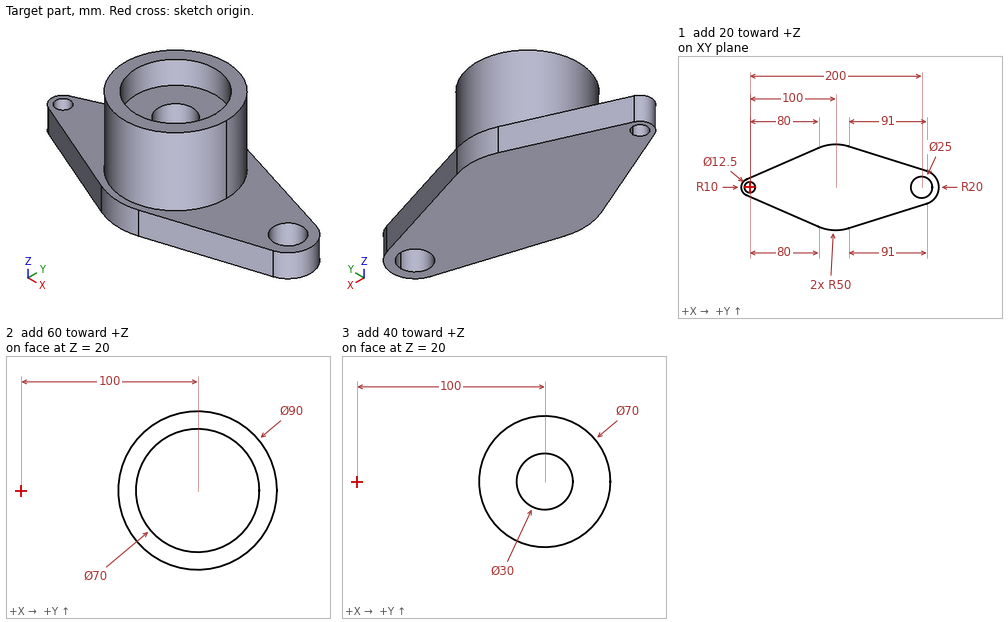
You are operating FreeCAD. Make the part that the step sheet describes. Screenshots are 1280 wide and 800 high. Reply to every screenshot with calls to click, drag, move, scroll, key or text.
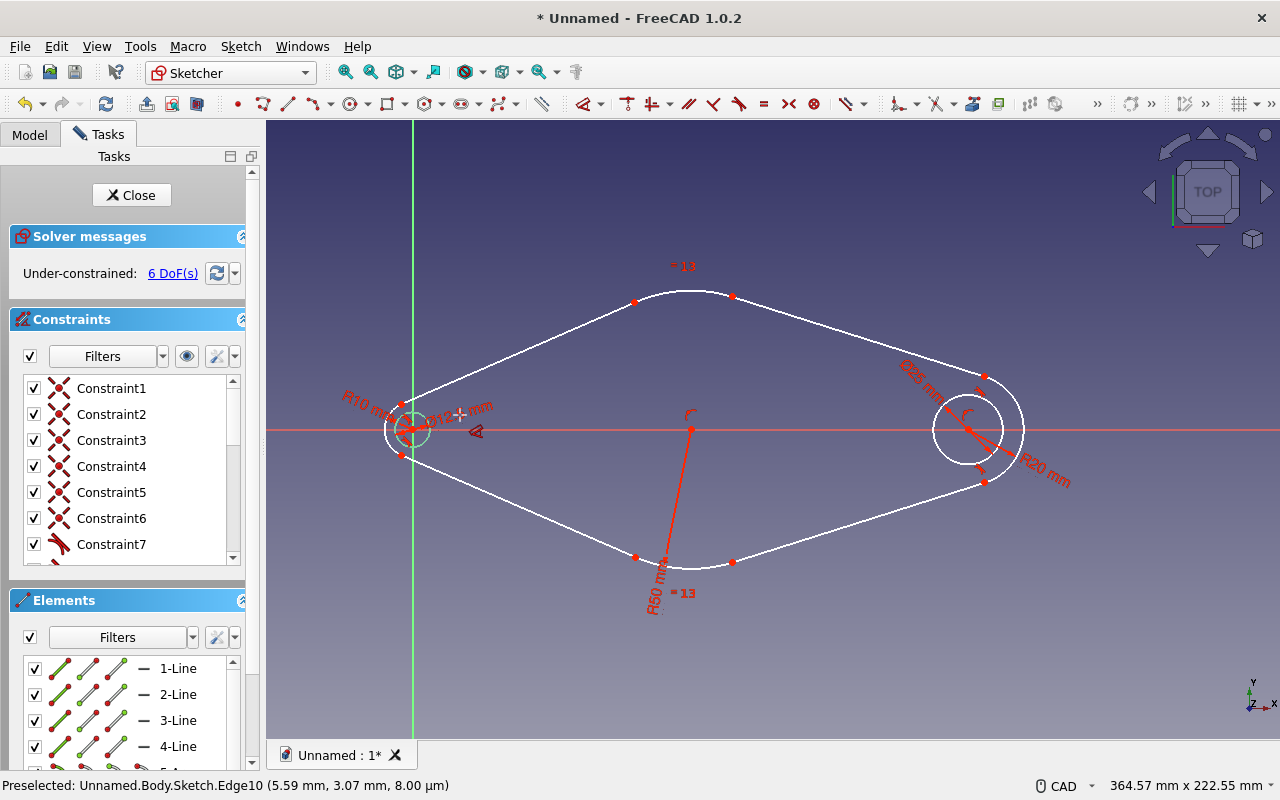
click(634, 303)
click(523, 269)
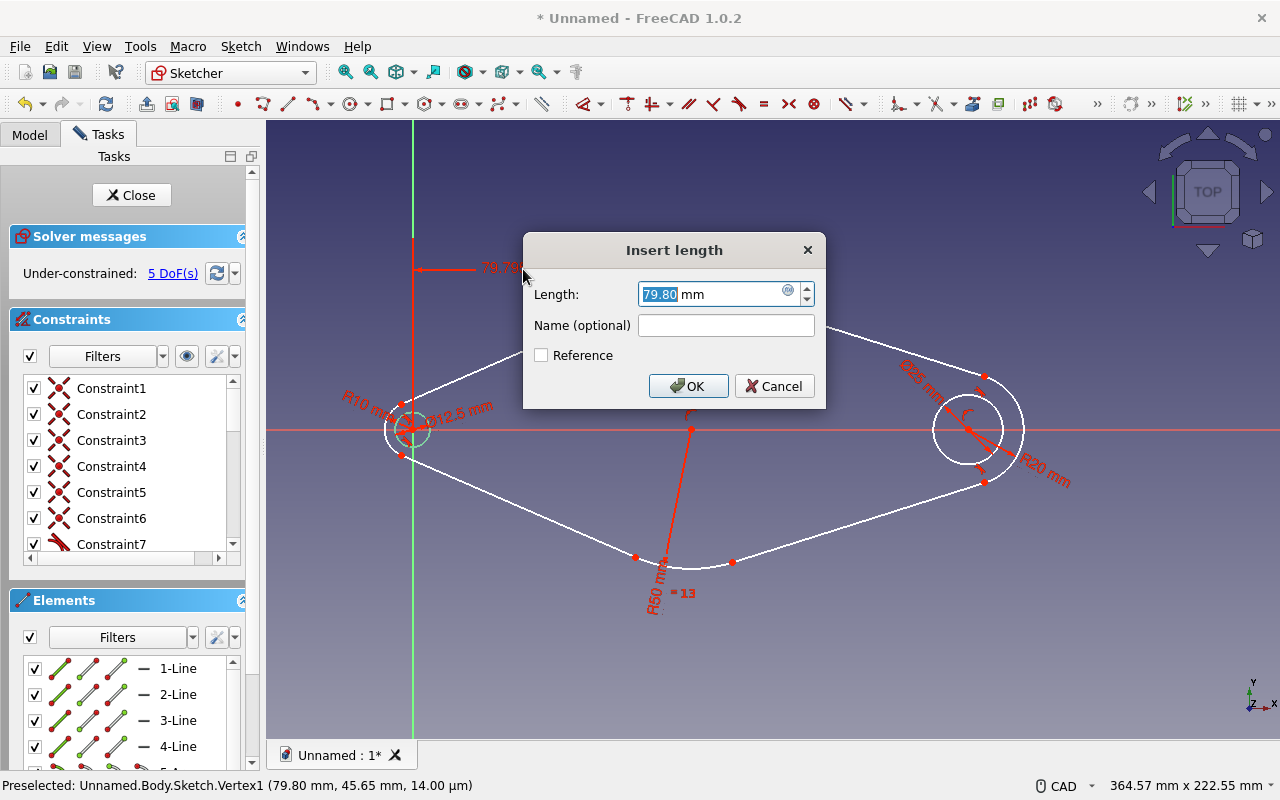
text(80)
key(Return)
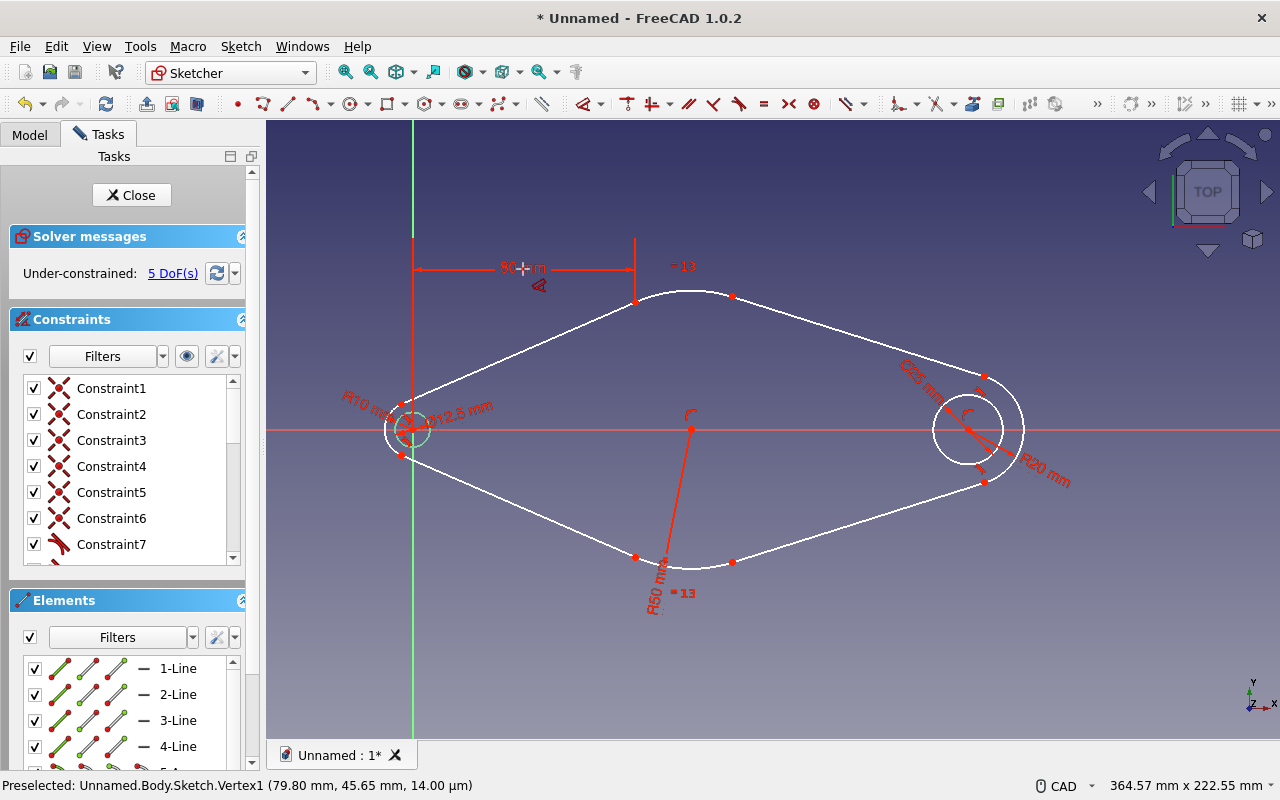
click(635, 557)
click(524, 591)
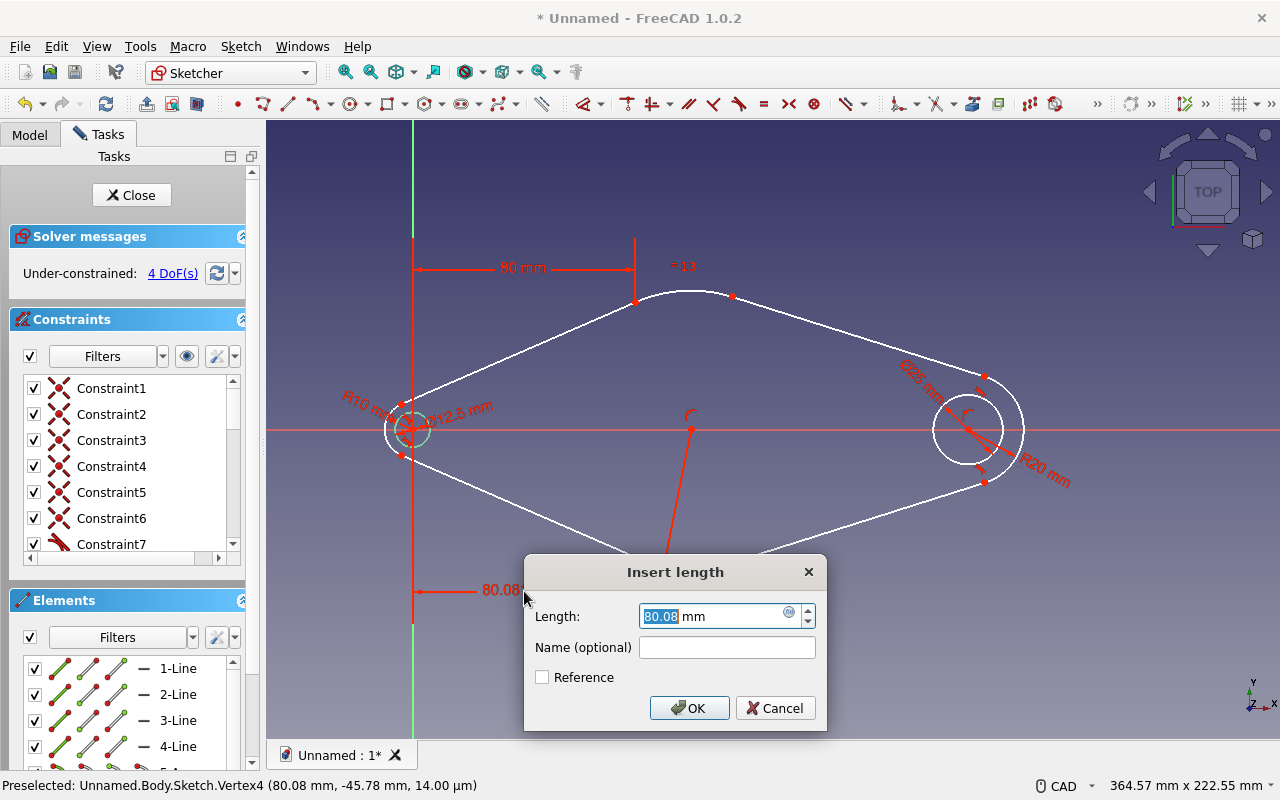
text(80)
key(Return)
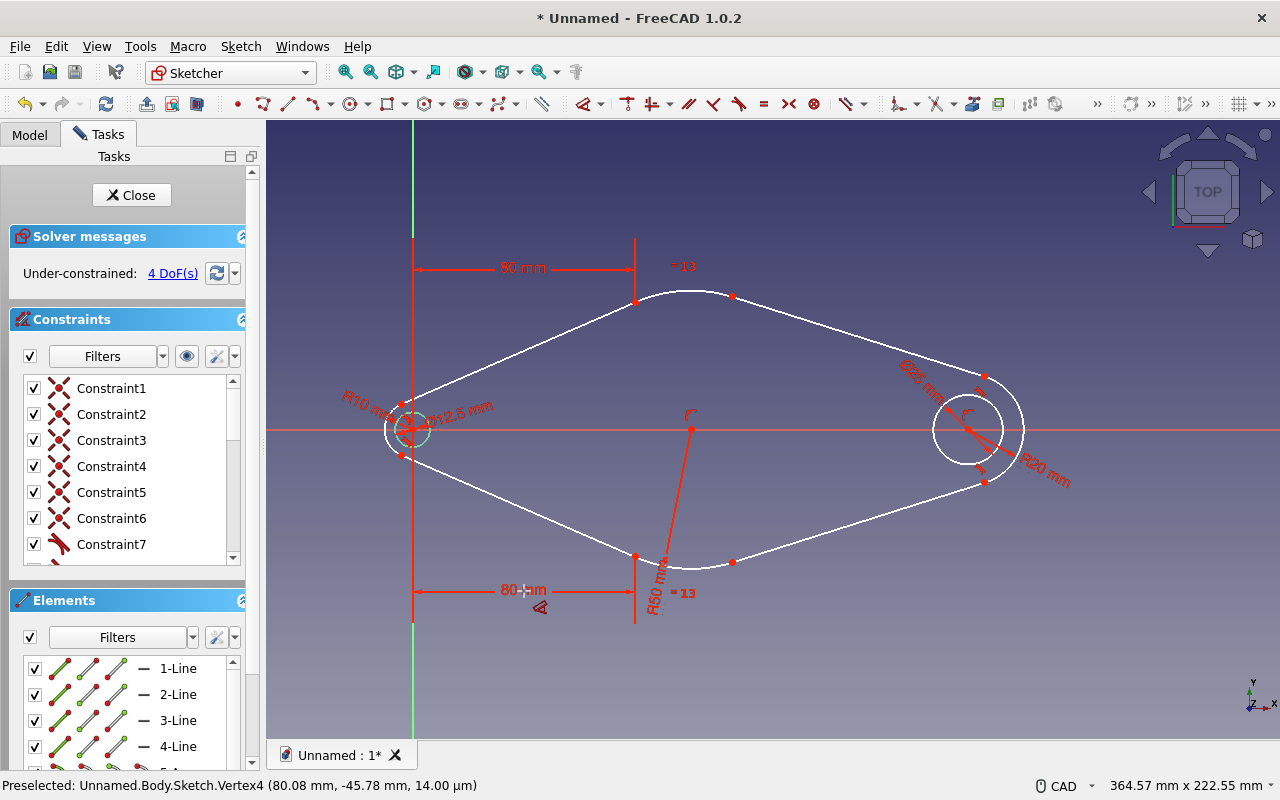
click(808, 539)
click(859, 597)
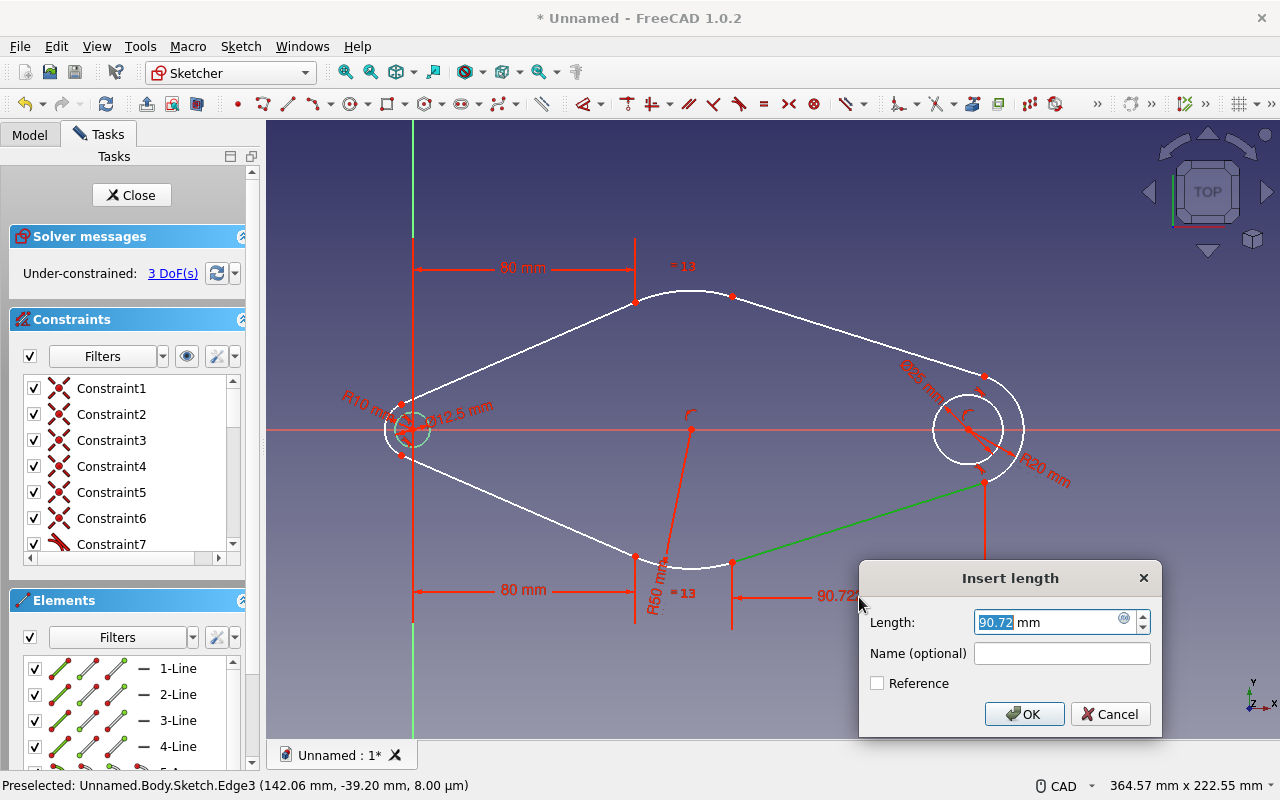
text(91)
key(Return)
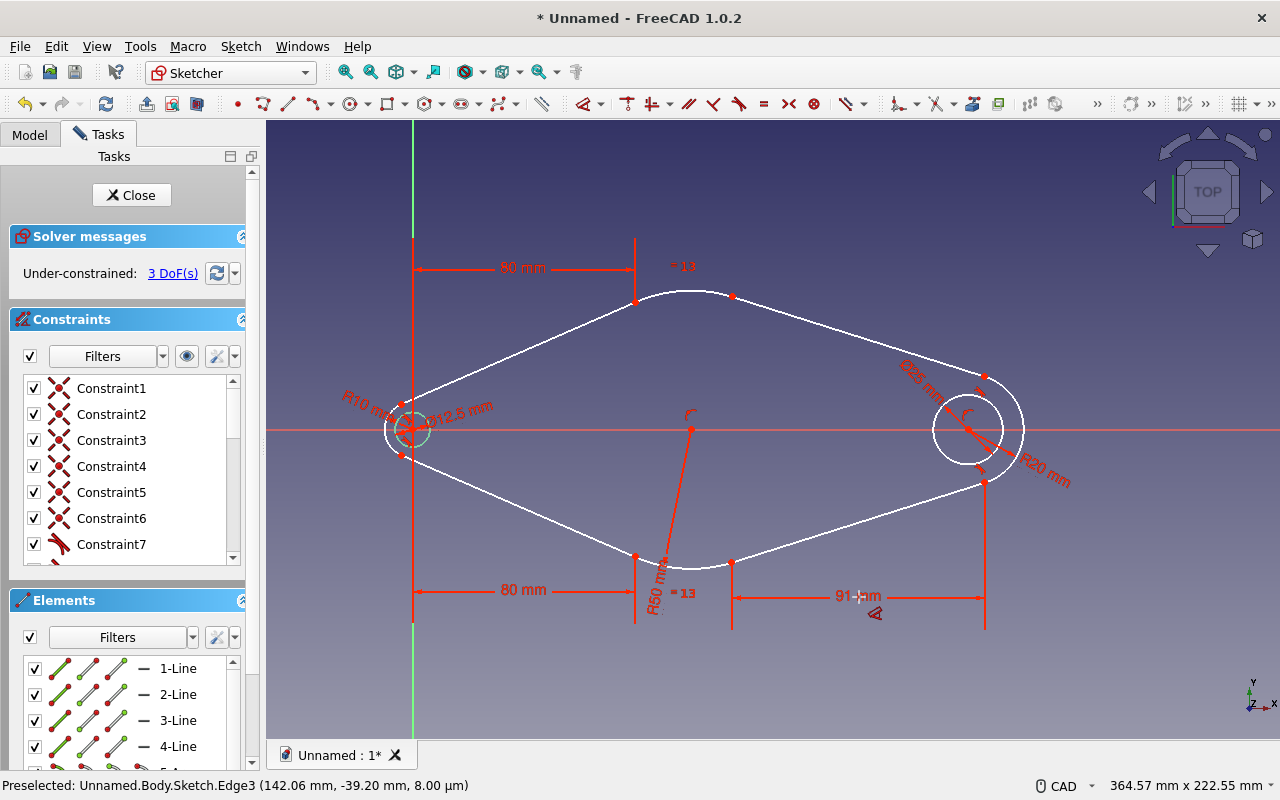
click(909, 353)
click(859, 263)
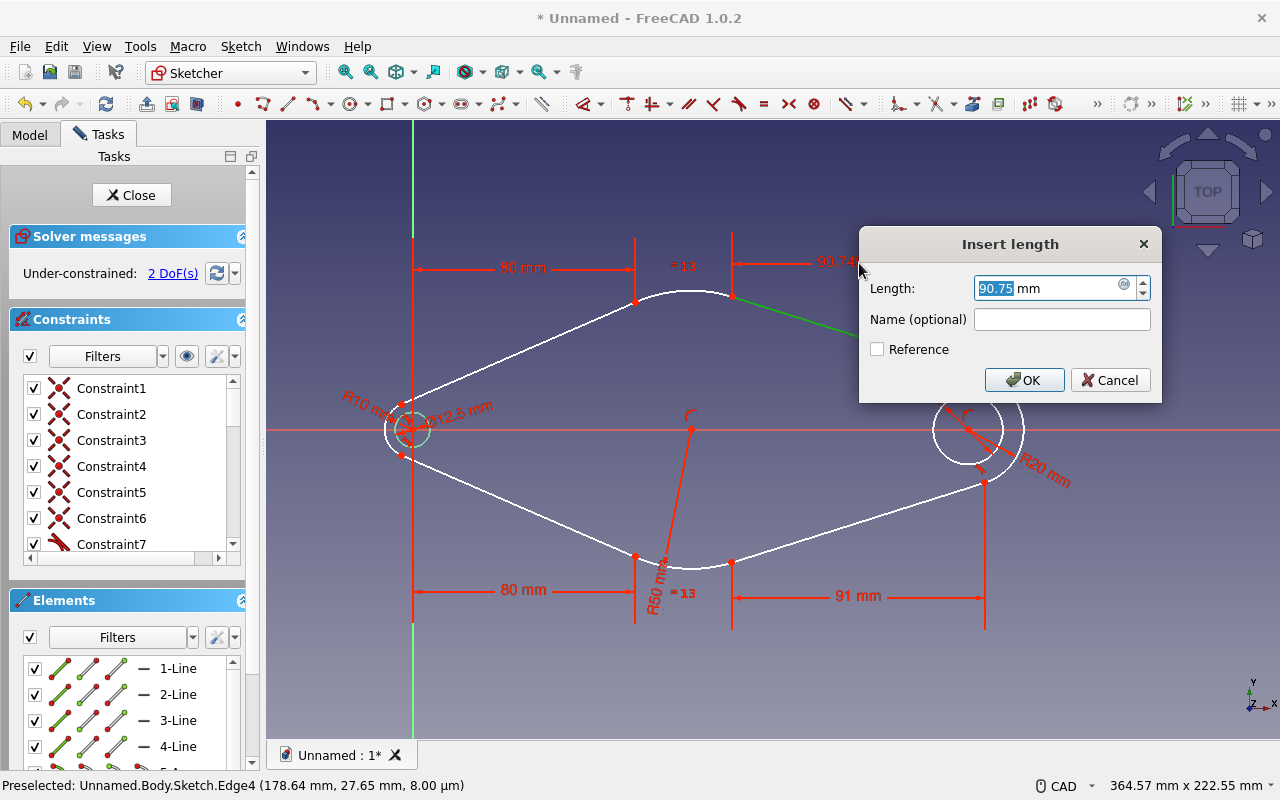
text(91)
key(Return)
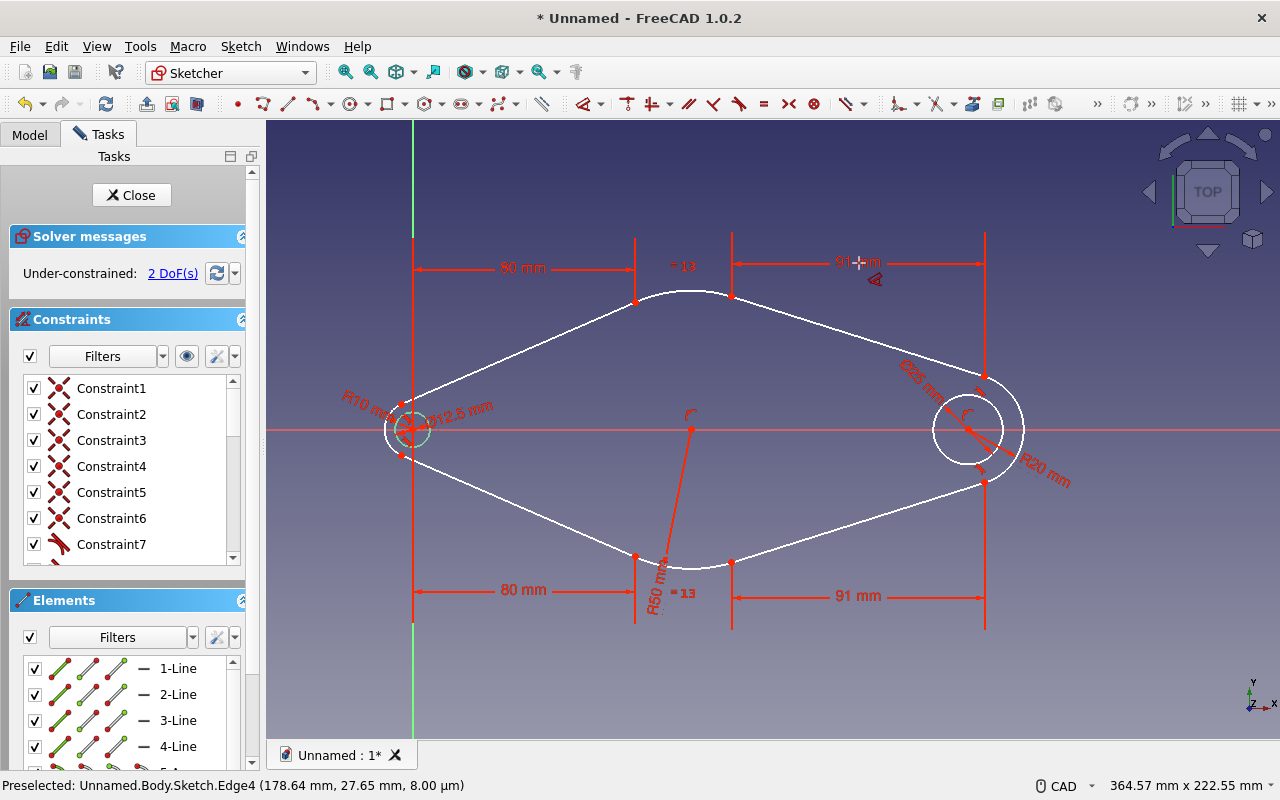
click(968, 430)
click(690, 464)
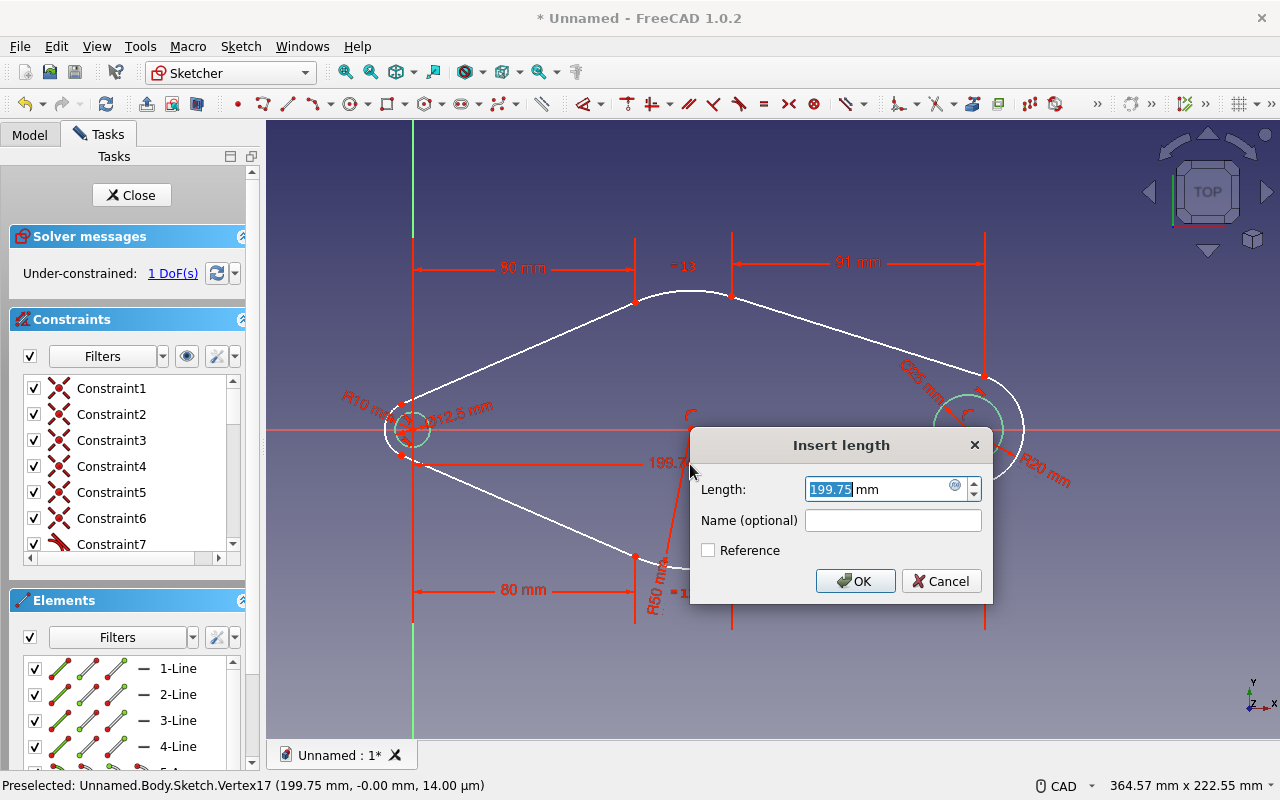
text(200)
key(Return)